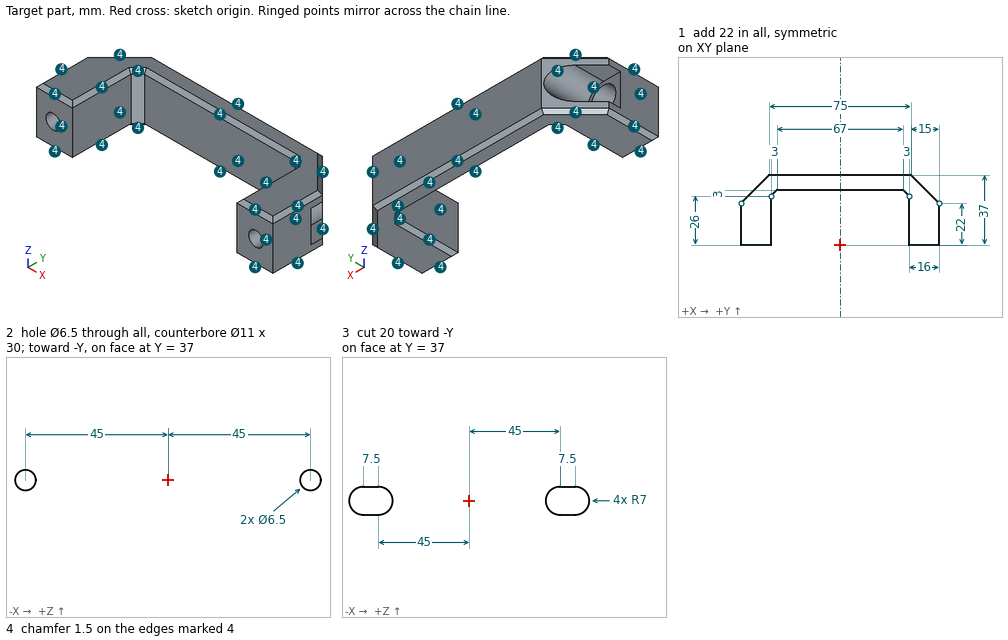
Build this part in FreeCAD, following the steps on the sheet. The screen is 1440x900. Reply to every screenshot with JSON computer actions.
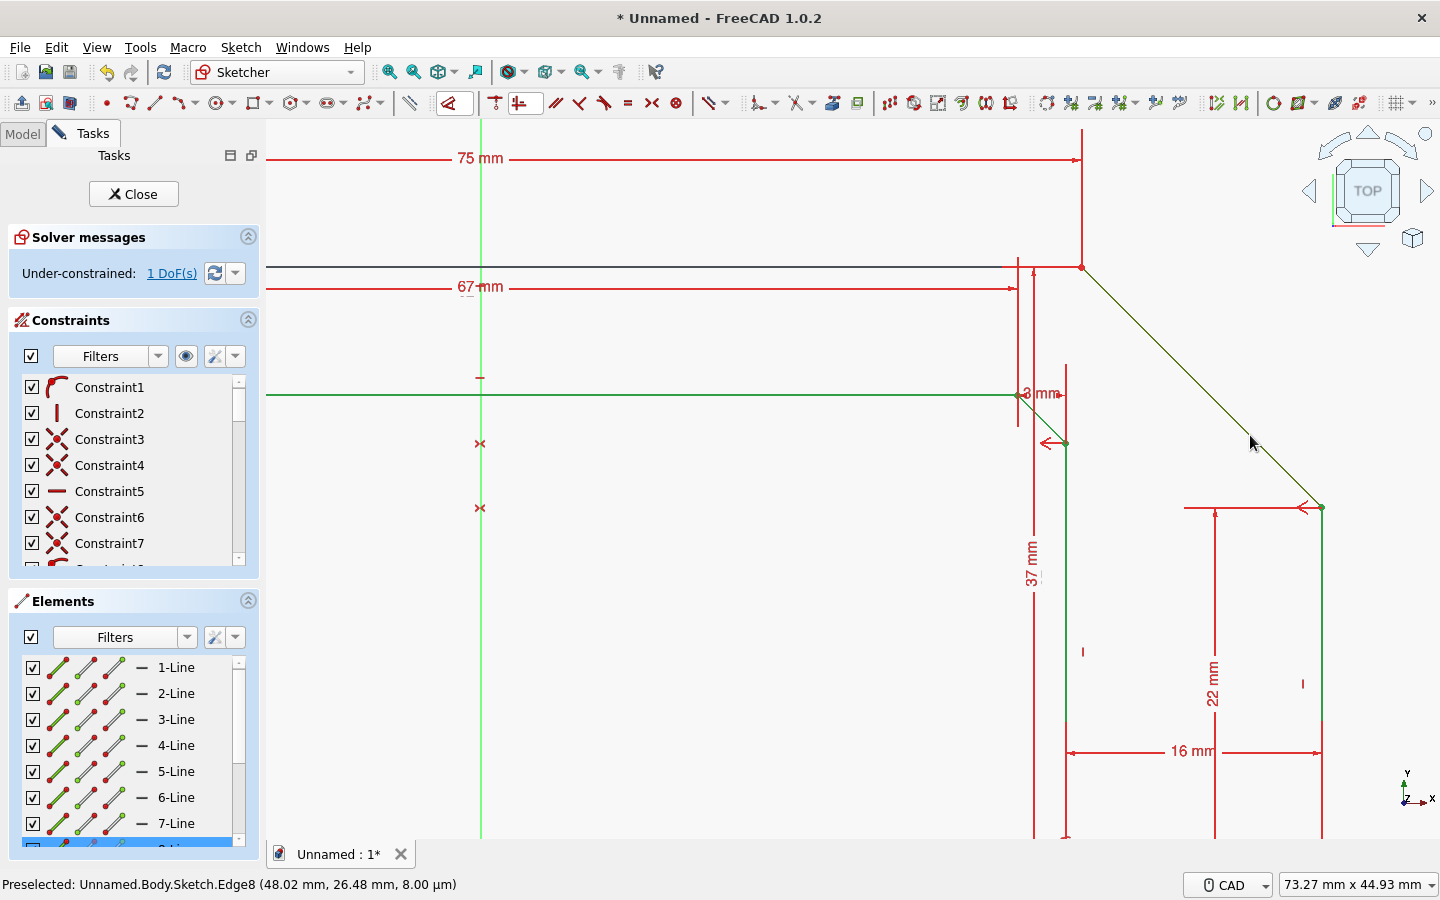
{"action": "key", "text": "l"}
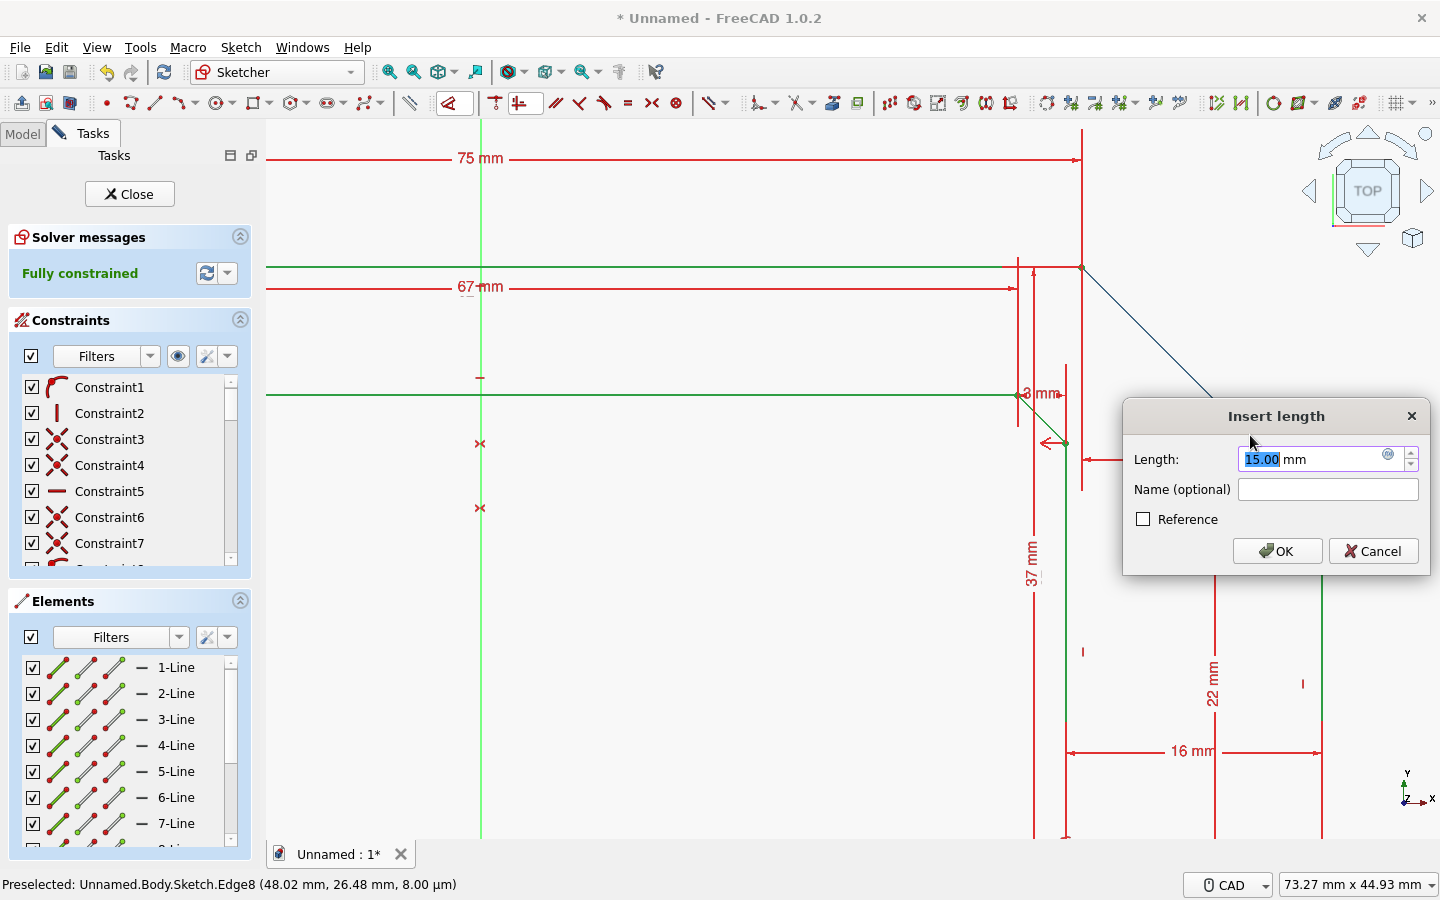
{"action": "type", "text": "15"}
{"action": "key", "text": "Return"}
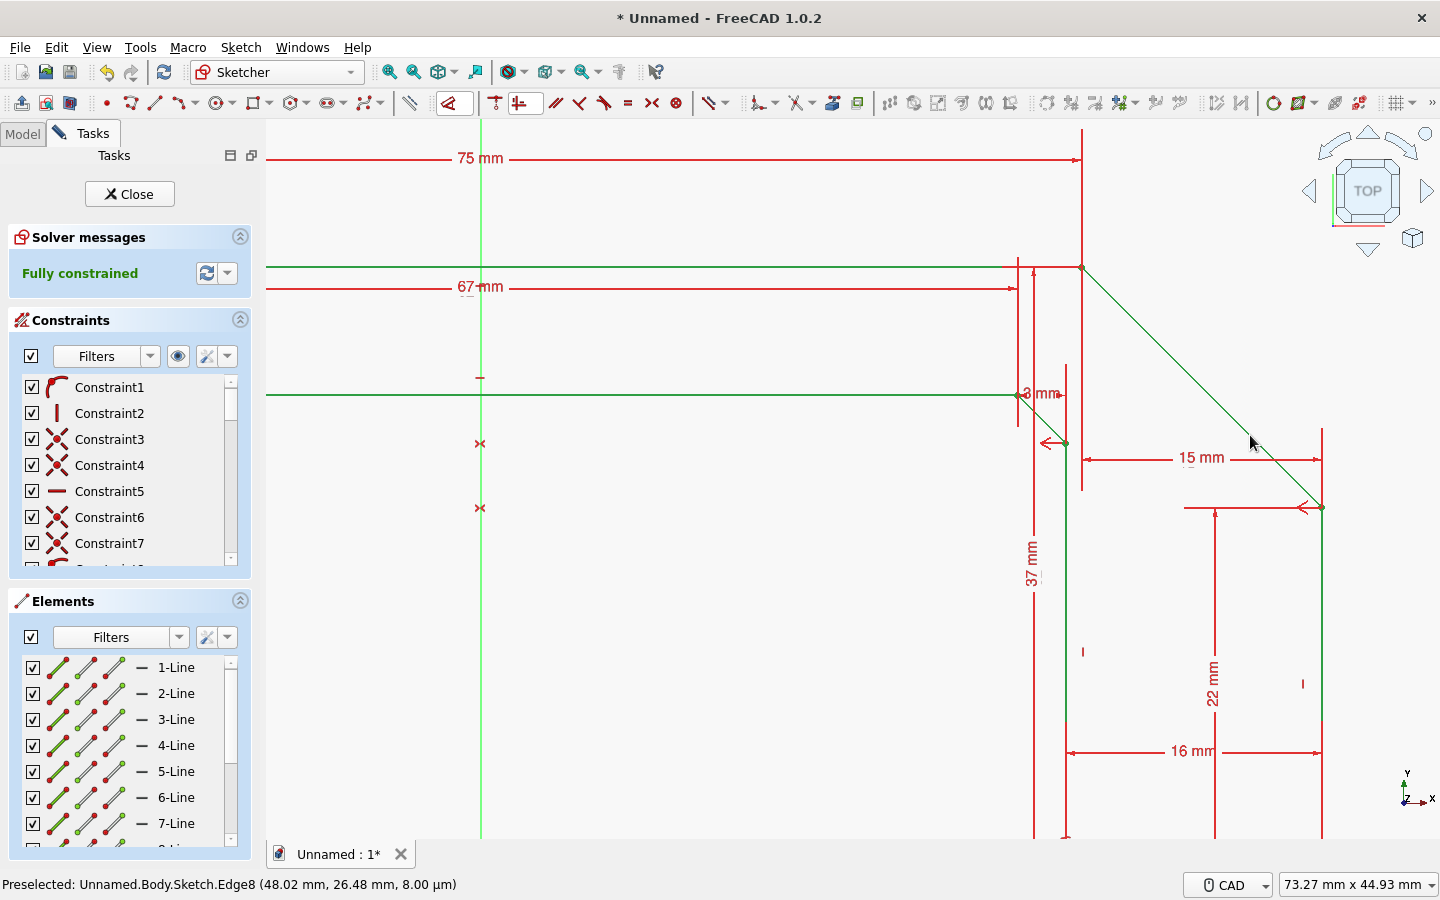
{"action": "left_click", "coordinate": [130, 194]}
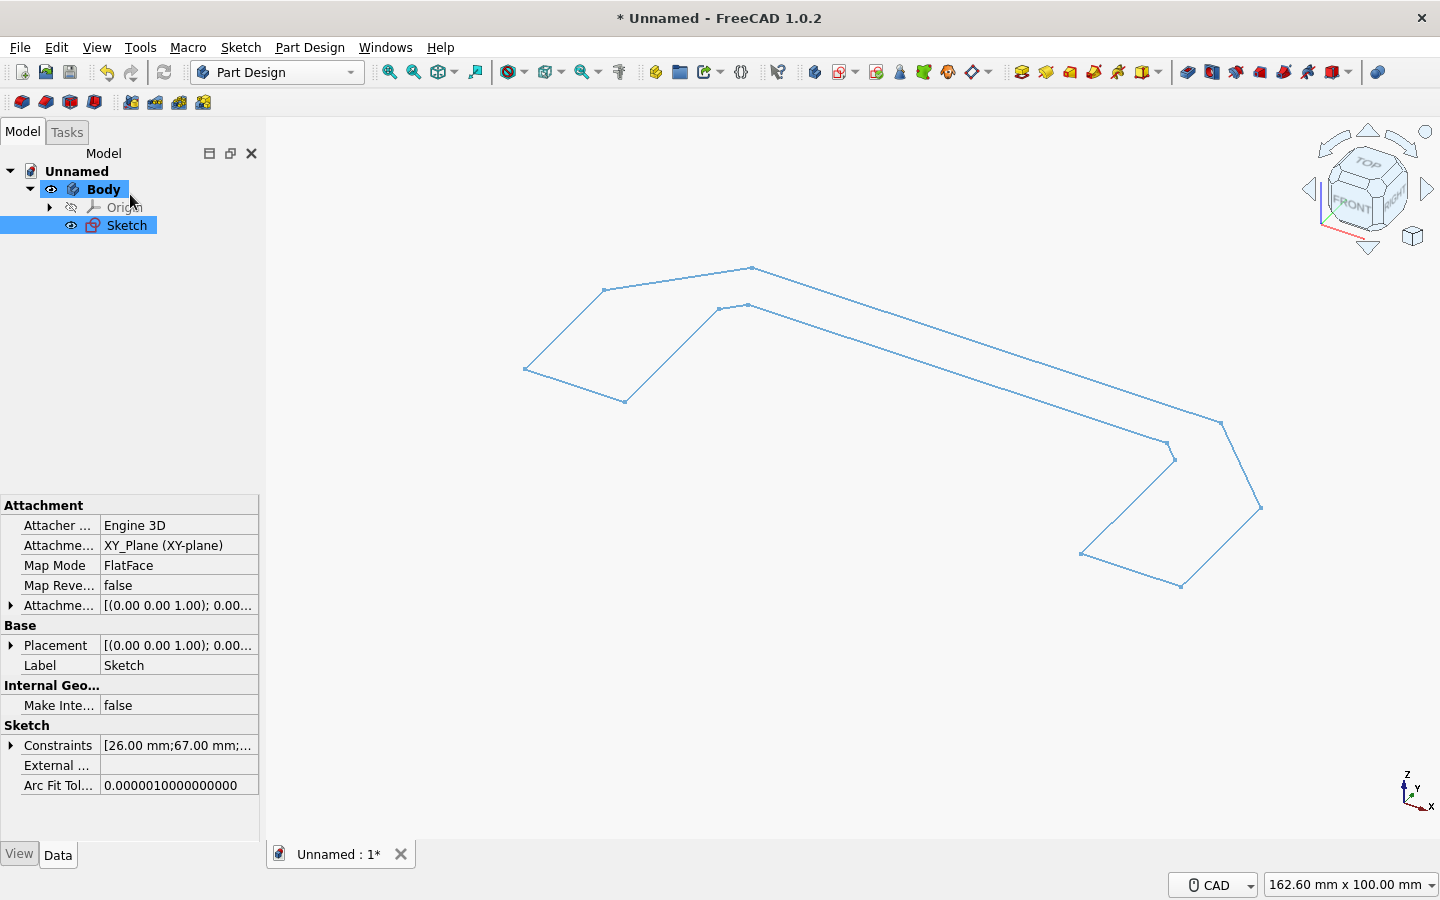
{"action": "left_click", "coordinate": [1022, 72]}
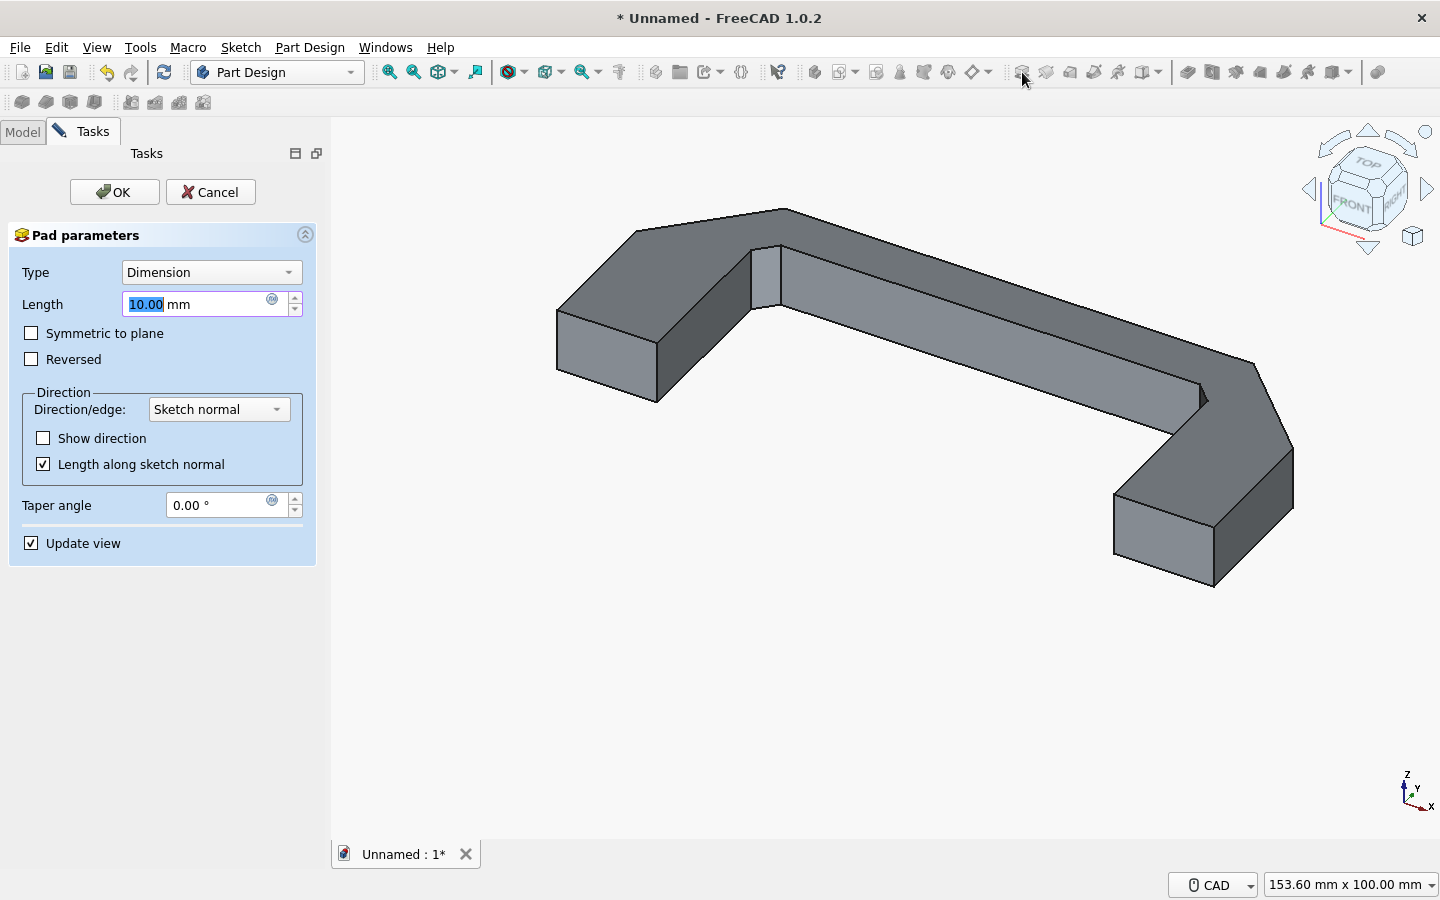
{"action": "type", "text": "22"}
{"action": "key", "text": "Tab"}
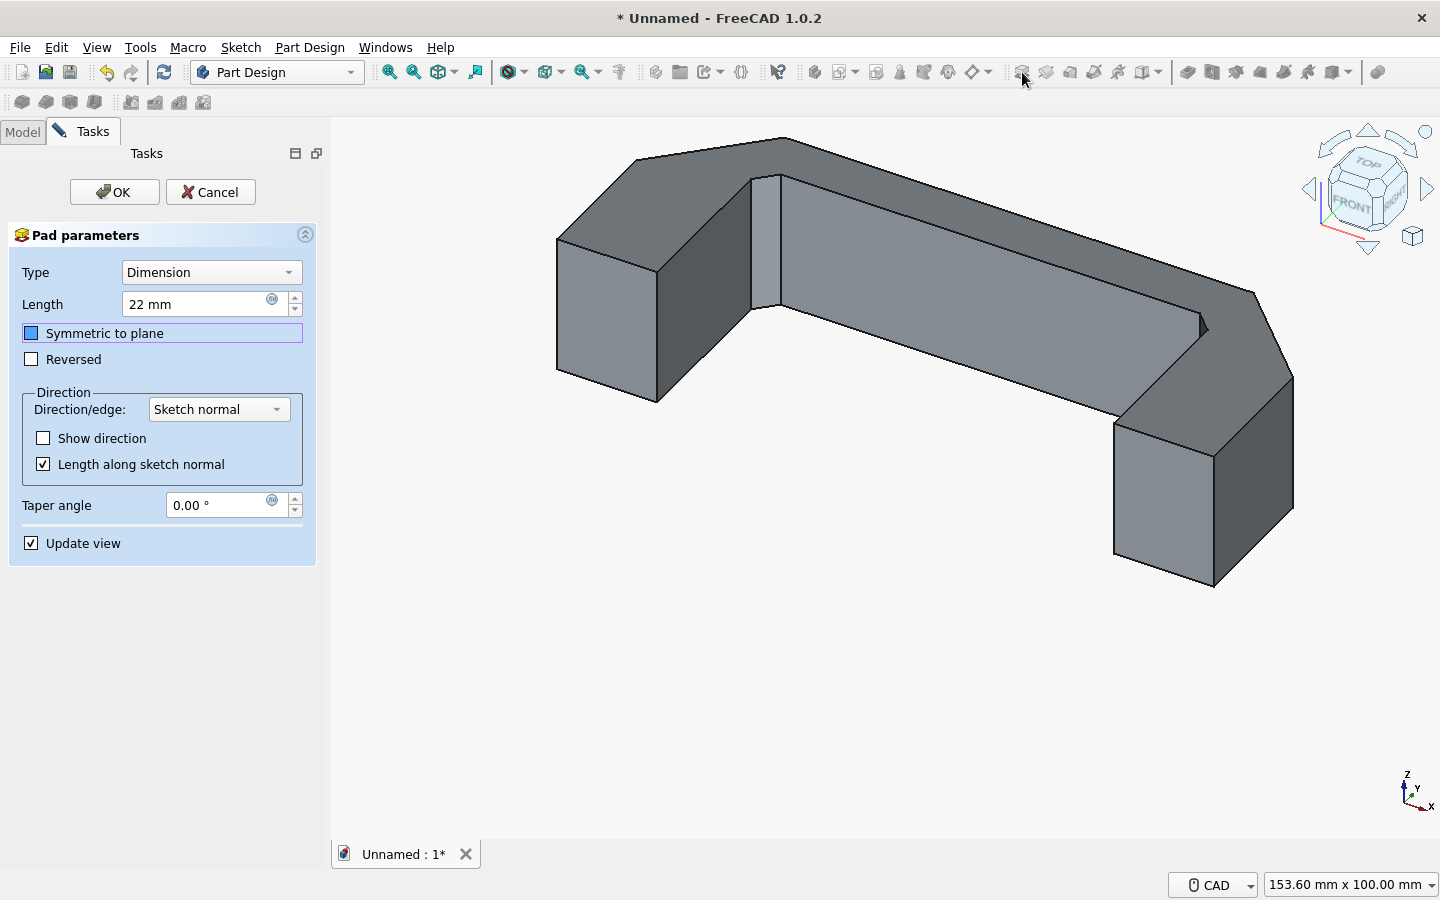
{"action": "left_click", "coordinate": [30, 333]}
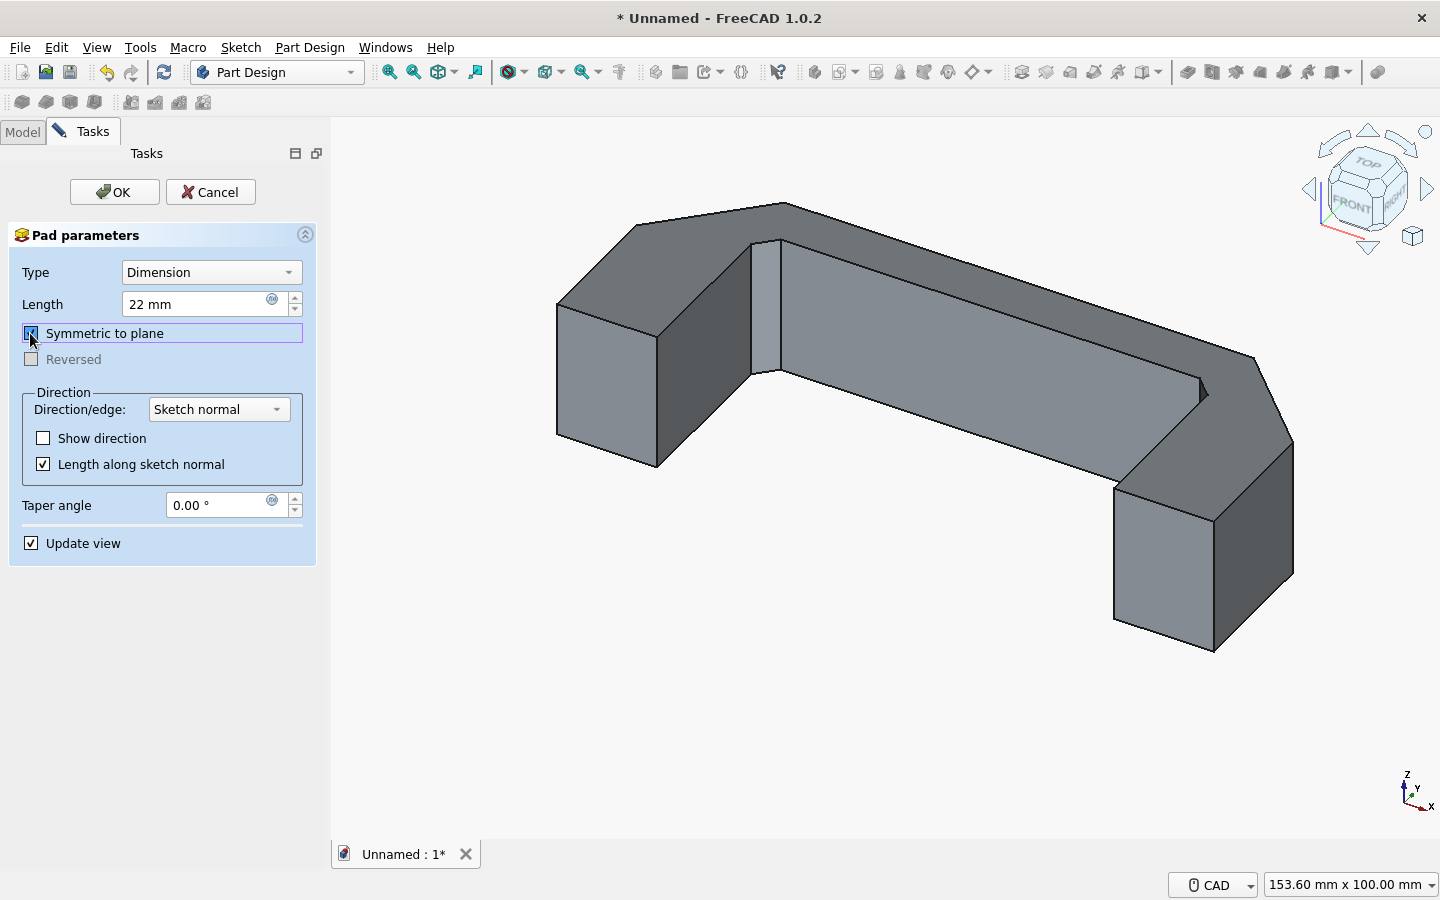
{"action": "left_click", "coordinate": [115, 192]}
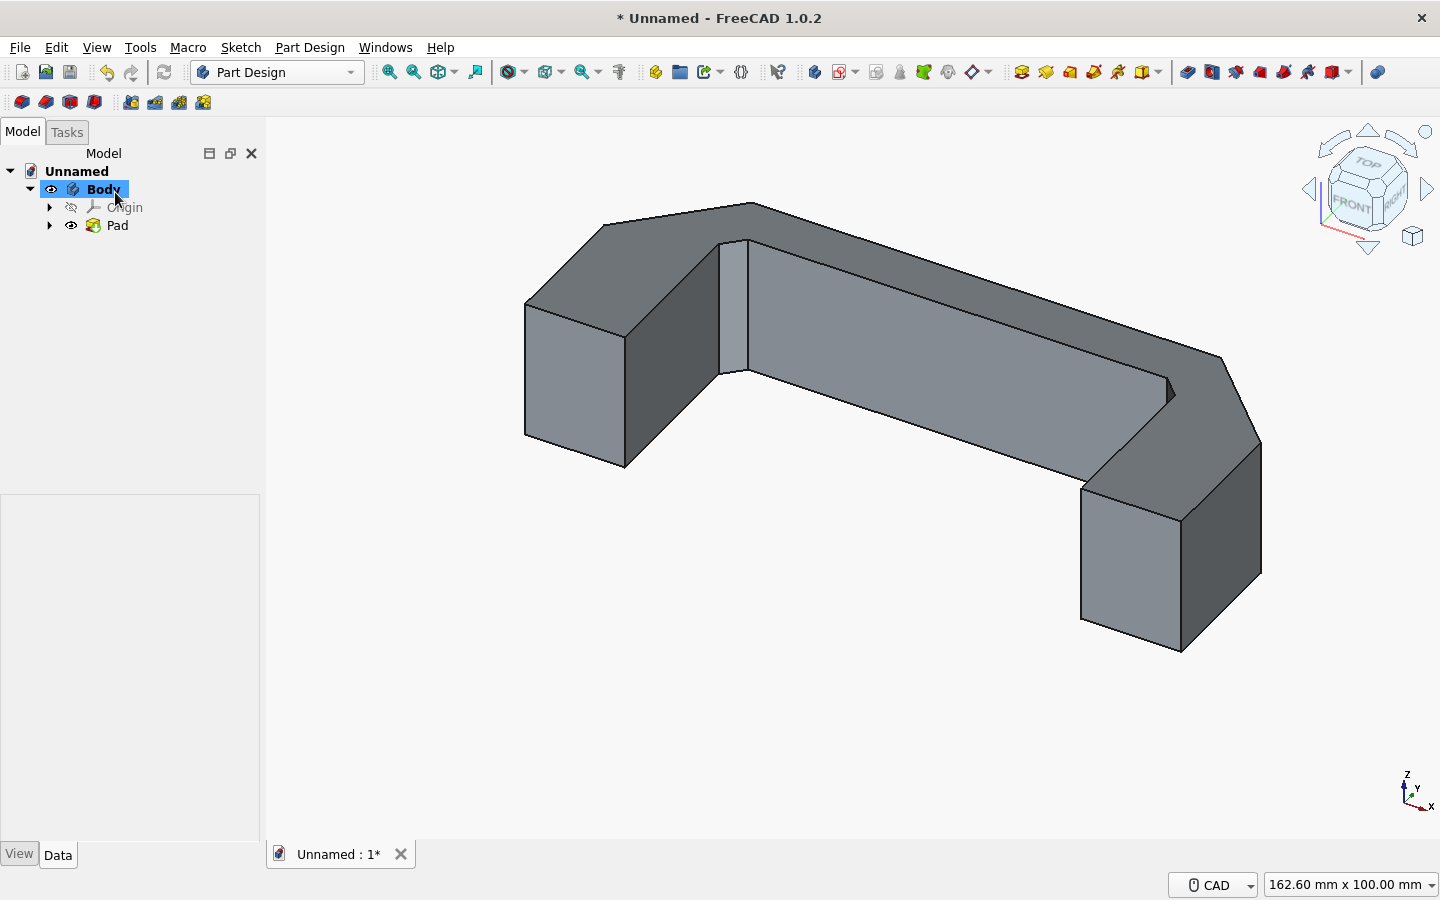
{"action": "key", "text": "4"}